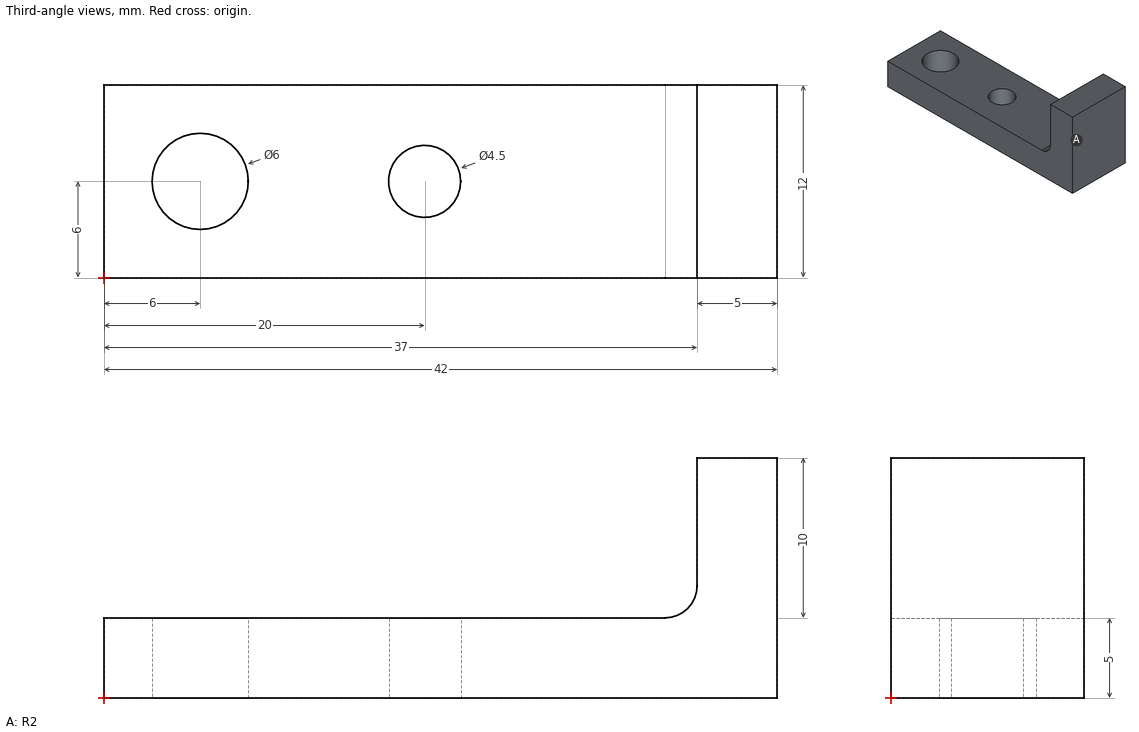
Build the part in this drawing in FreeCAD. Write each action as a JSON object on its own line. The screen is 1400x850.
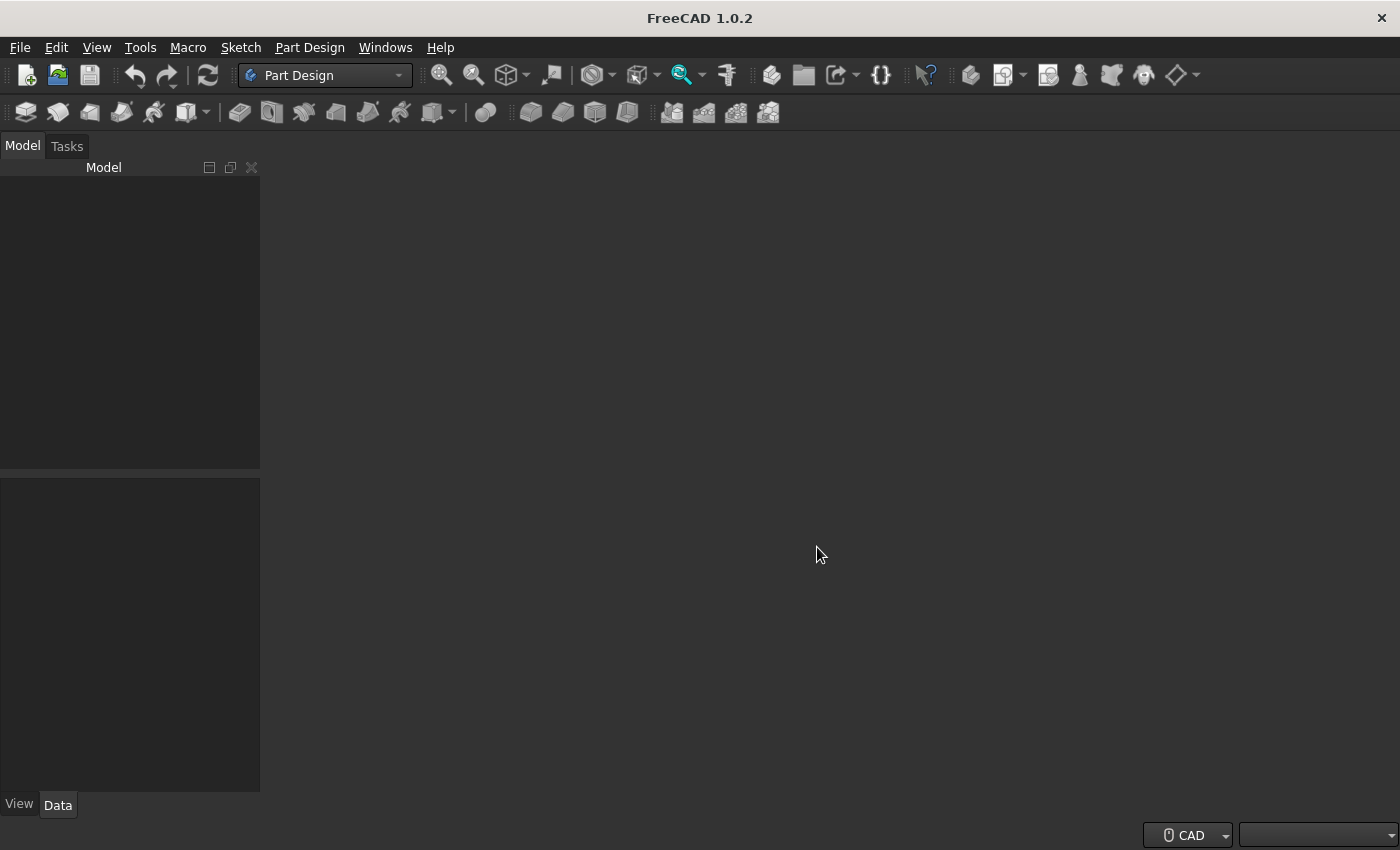
{"action": "key", "text": "ctrl+n"}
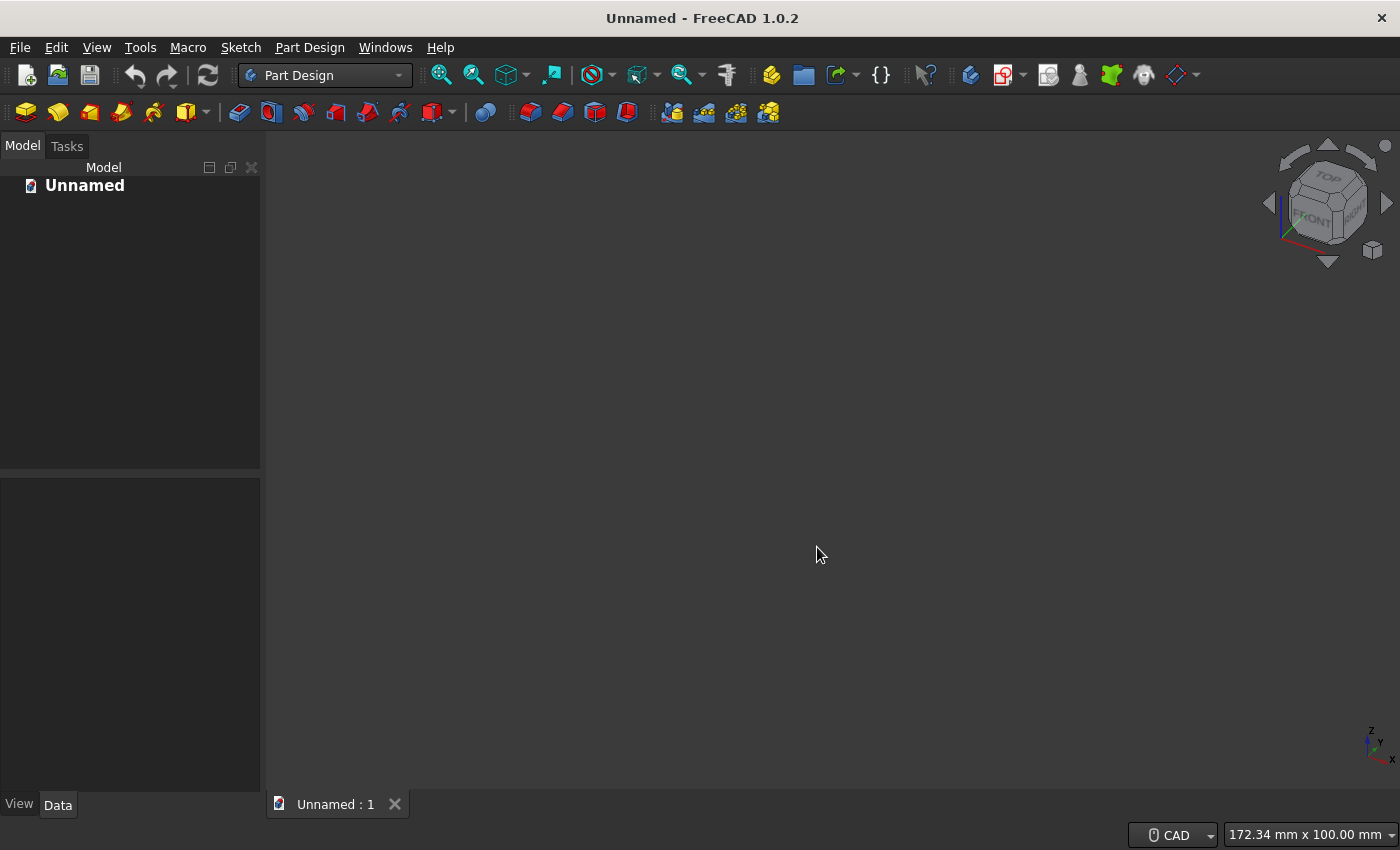
{"action": "left_click", "coordinate": [1004, 76]}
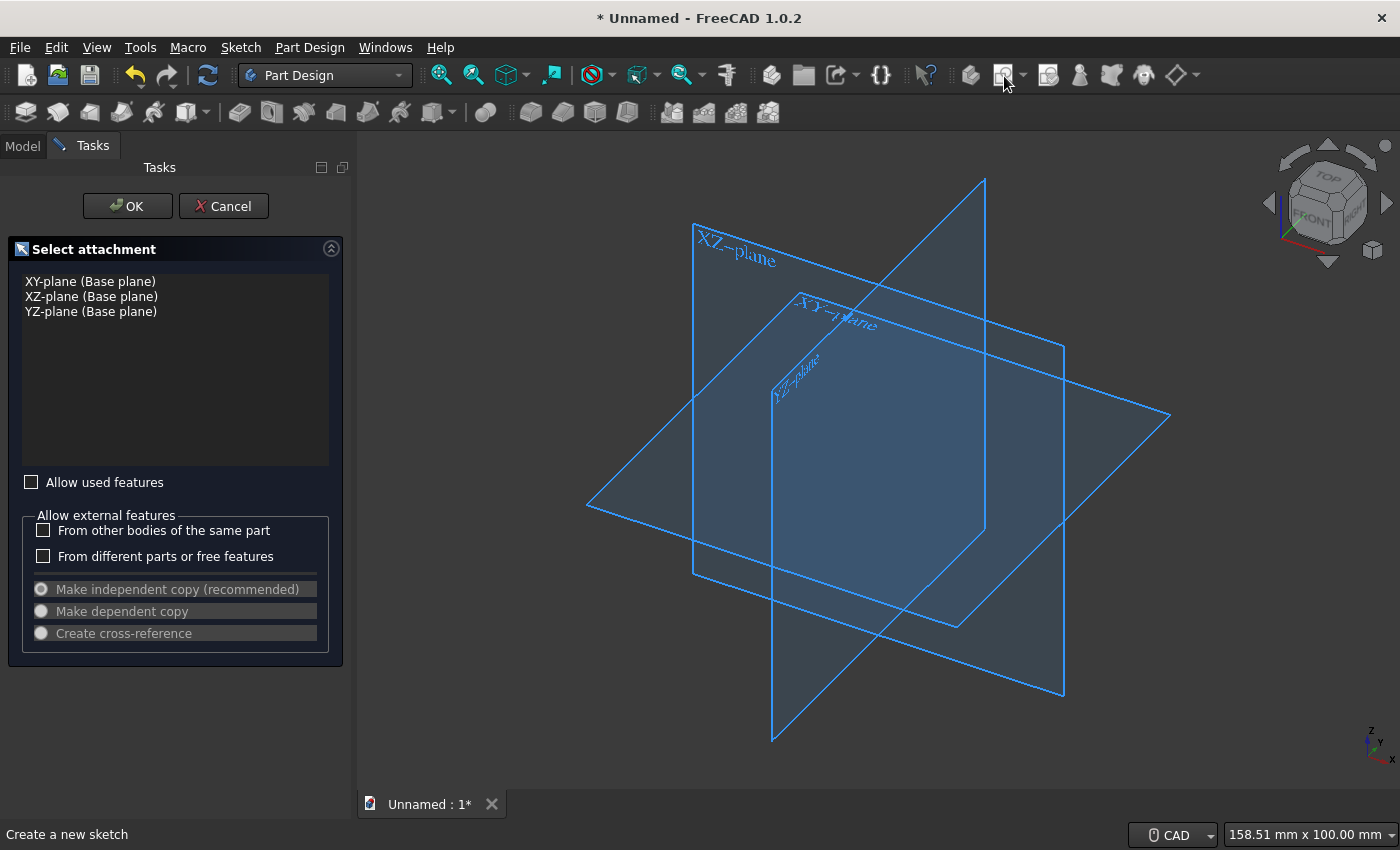
{"action": "left_click", "coordinate": [82, 282]}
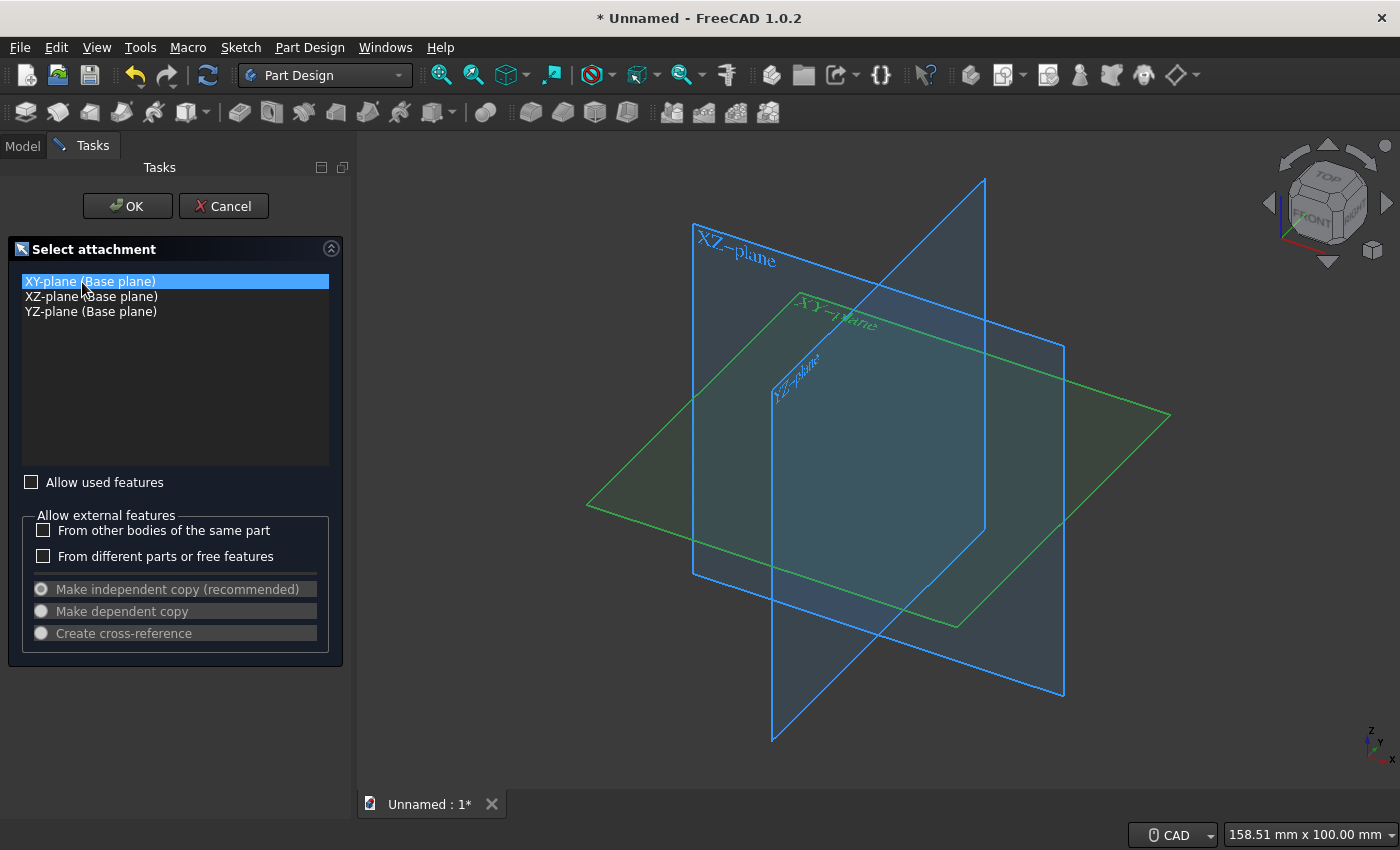
{"action": "left_click", "coordinate": [128, 206]}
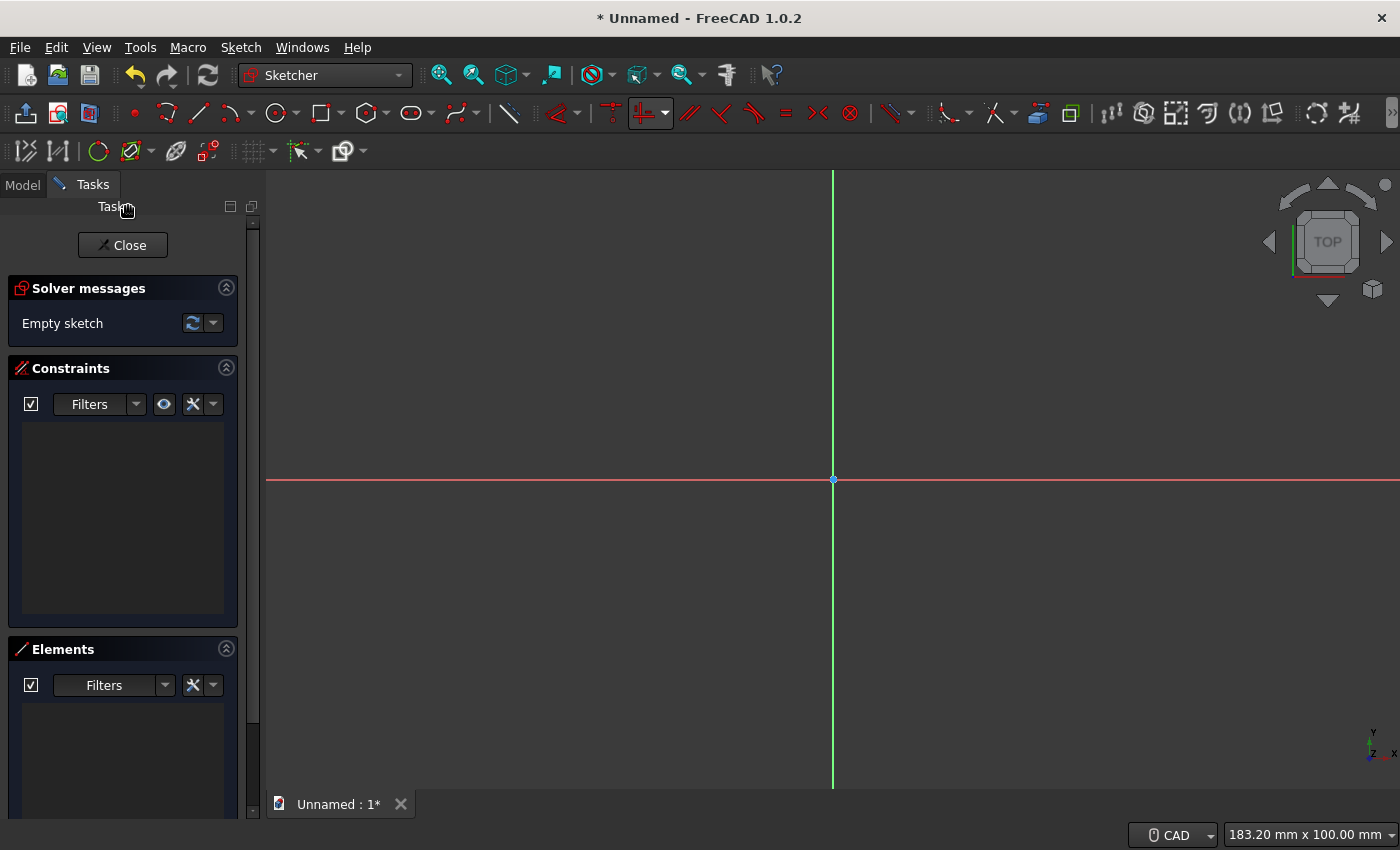
{"action": "scroll", "coordinate": [1079, 421], "scroll_direction": "up", "scroll_amount": 5}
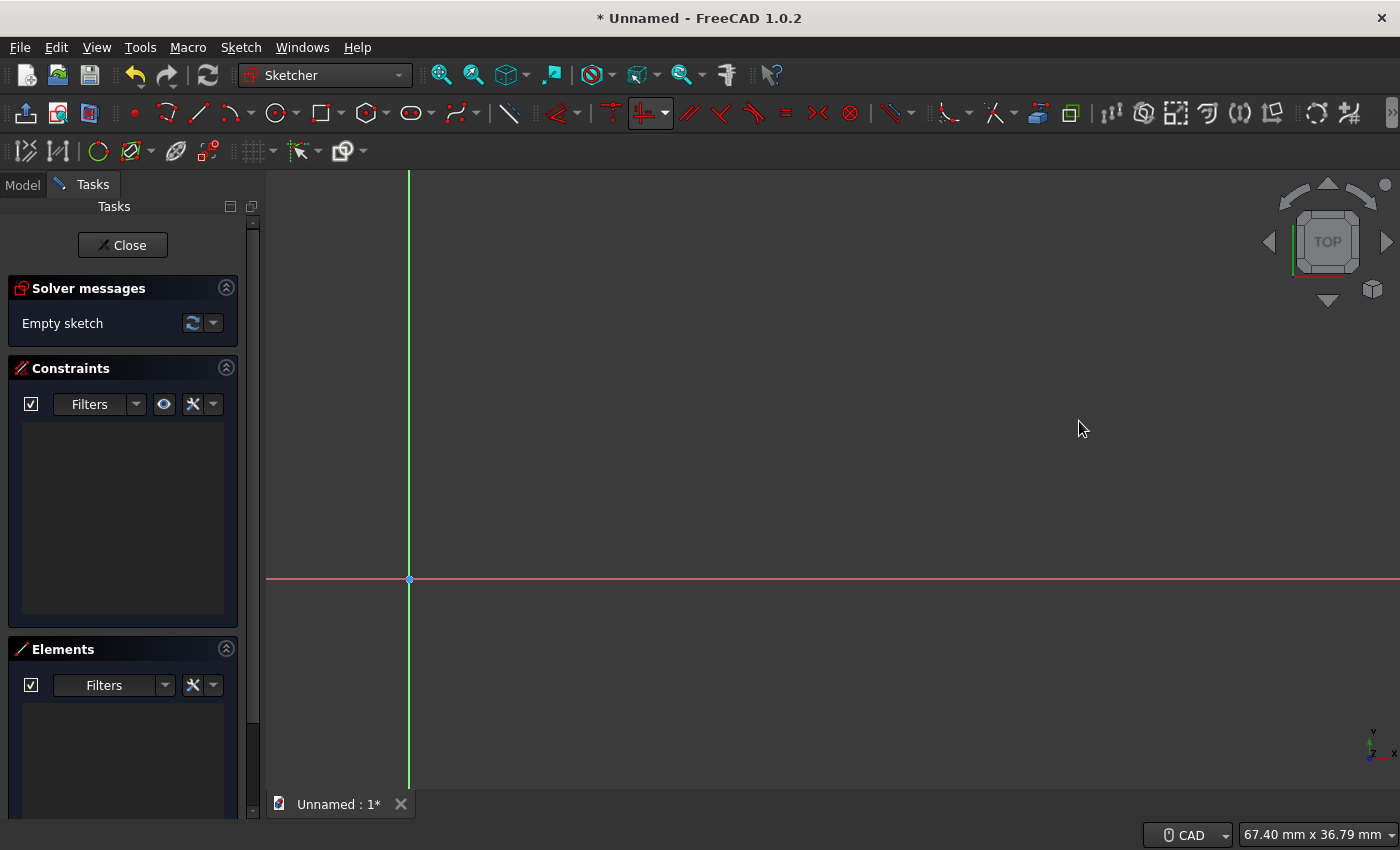
{"action": "left_click", "coordinate": [322, 114]}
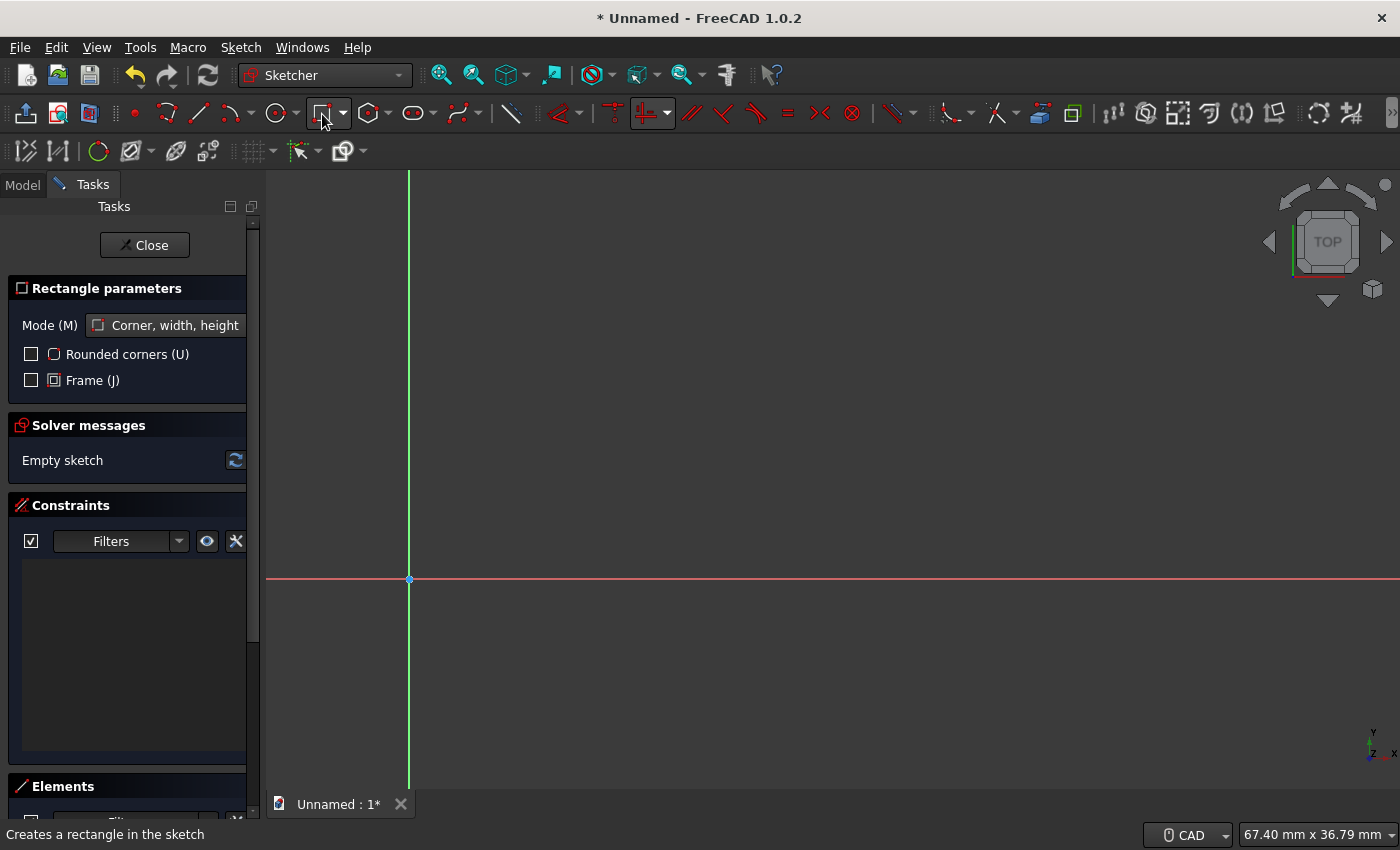
{"action": "left_click", "coordinate": [409, 579]}
{"action": "mouse_move", "coordinate": [1116, 377]}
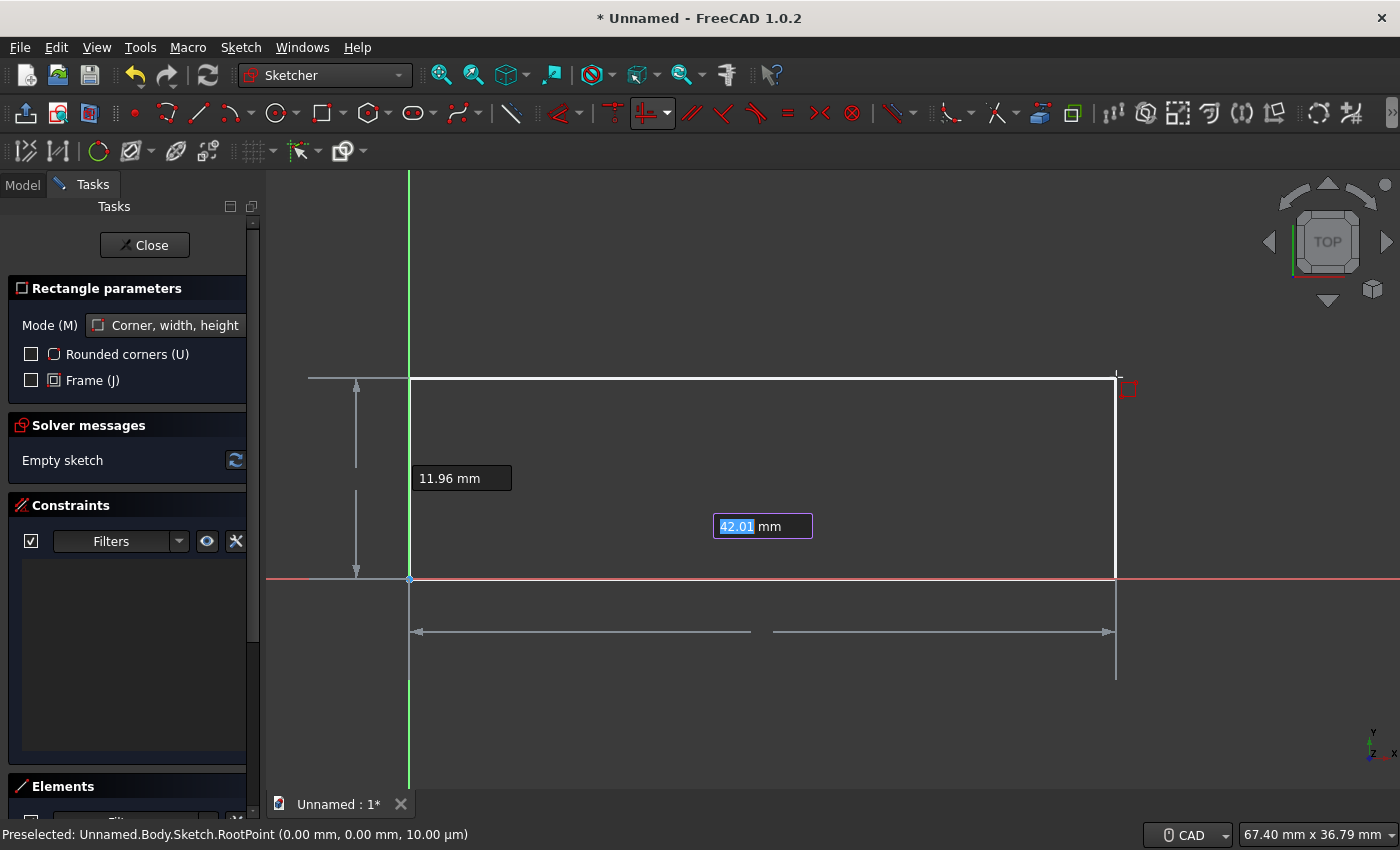
{"action": "type", "text": "42"}
{"action": "key", "text": "Tab"}
{"action": "type", "text": "12"}
{"action": "key", "text": "Return"}